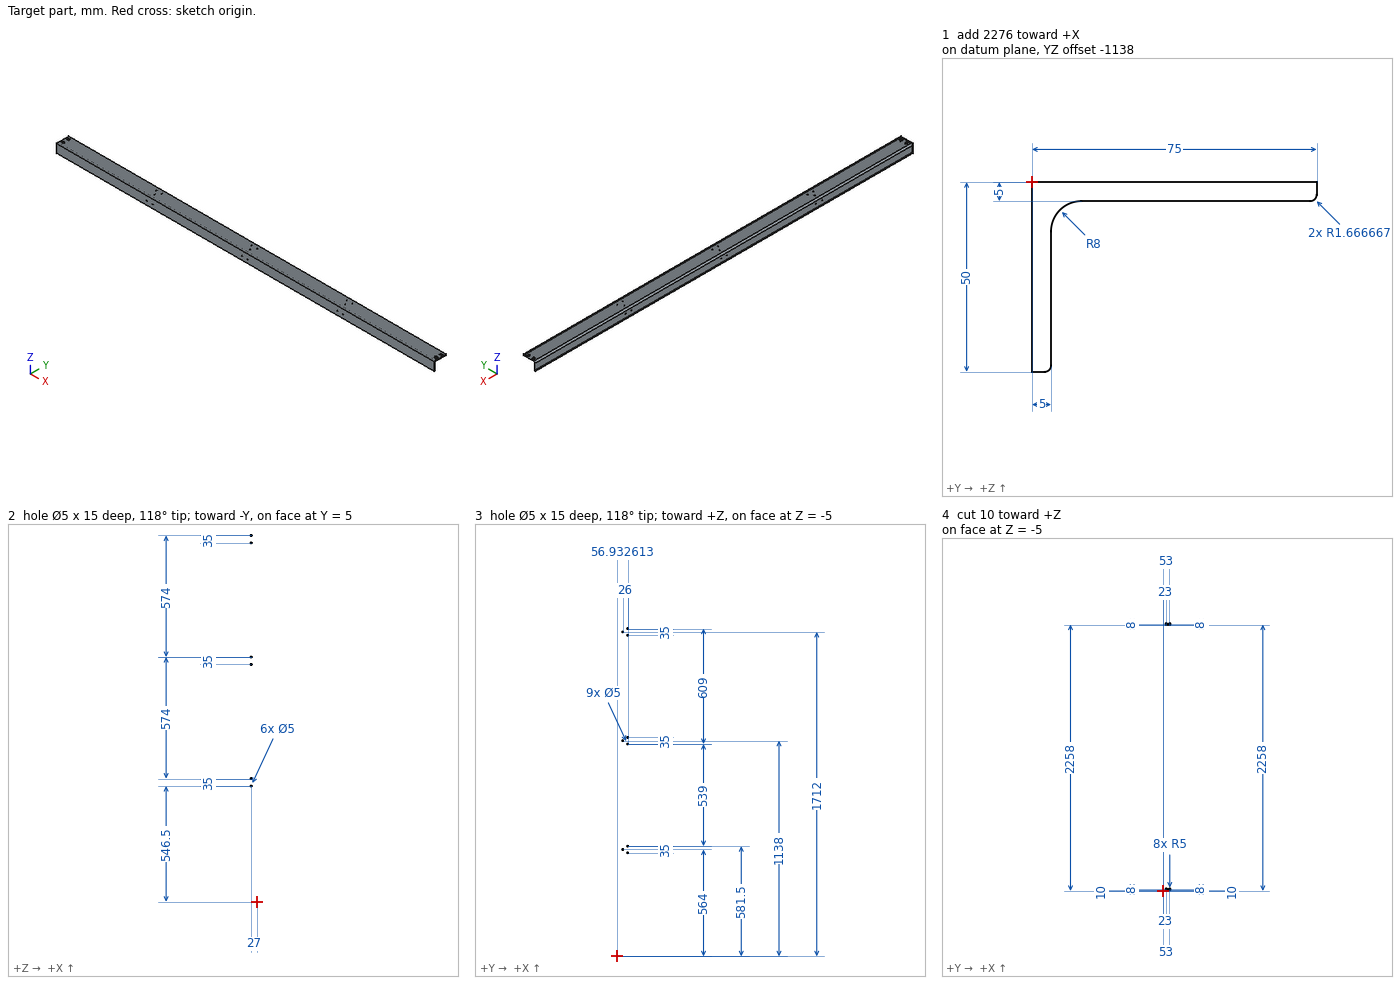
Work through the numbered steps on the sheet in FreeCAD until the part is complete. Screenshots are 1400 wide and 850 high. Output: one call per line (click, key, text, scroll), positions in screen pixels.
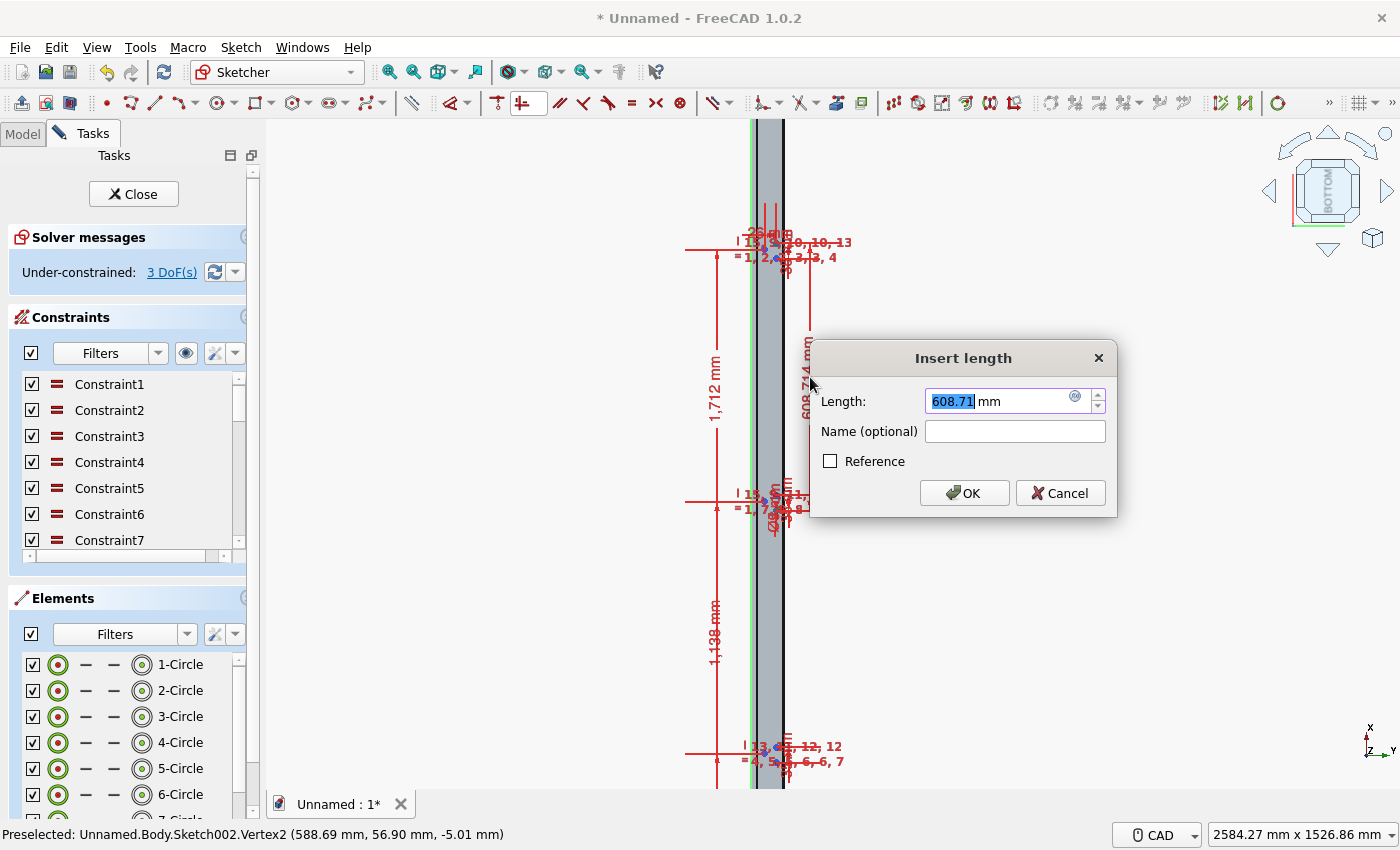
text(609)
key(Return)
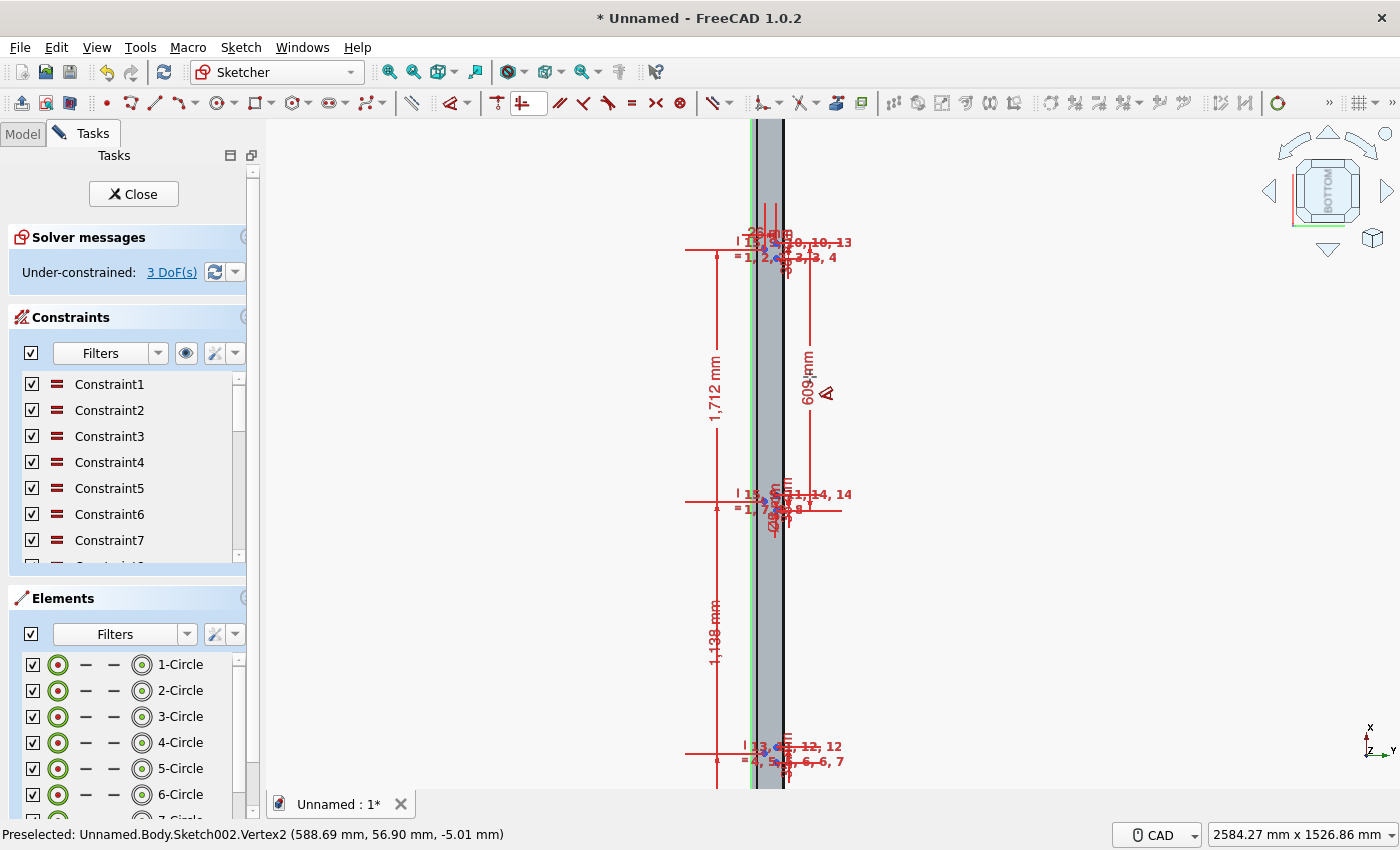
click(776, 511)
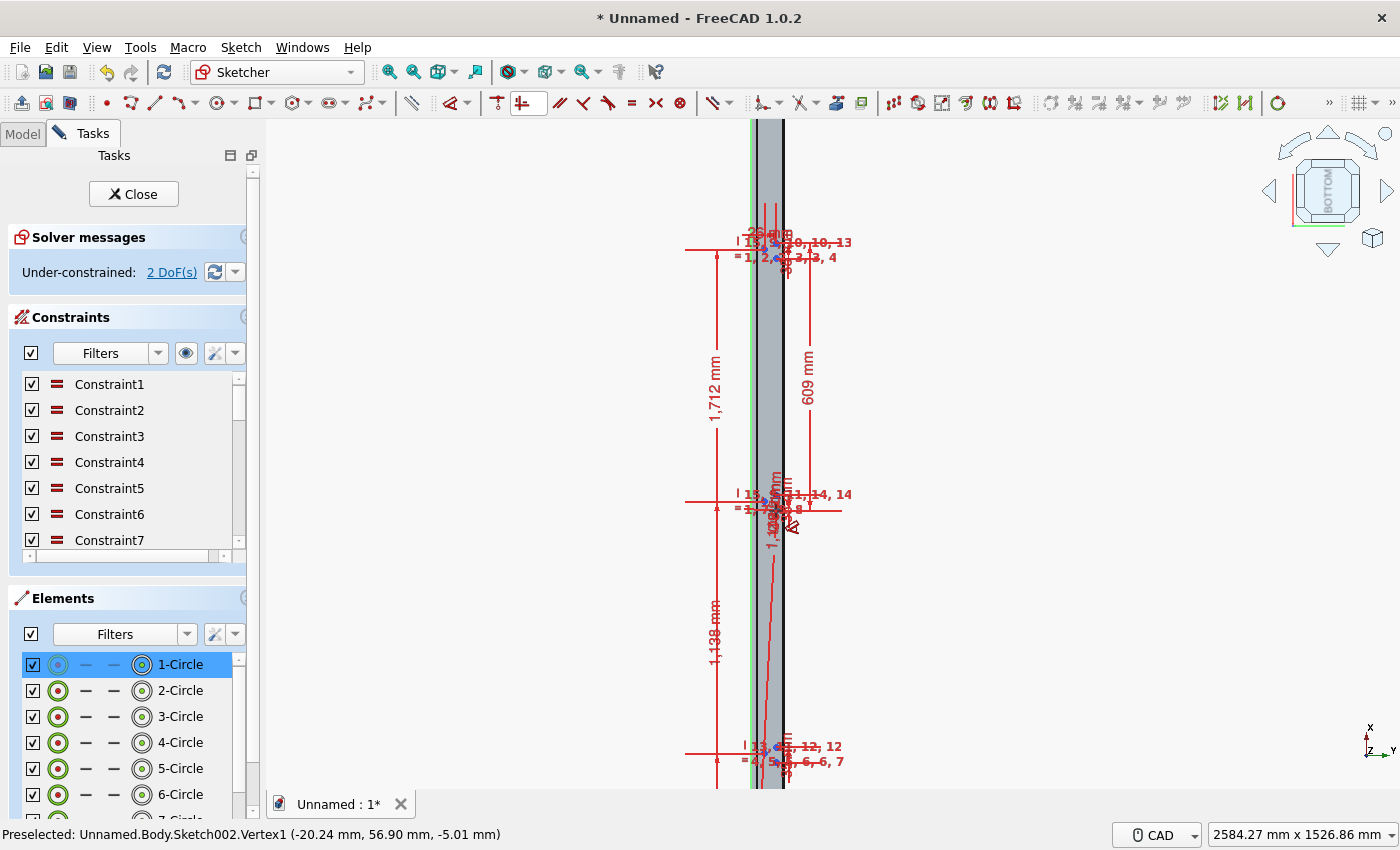
click(776, 747)
click(810, 629)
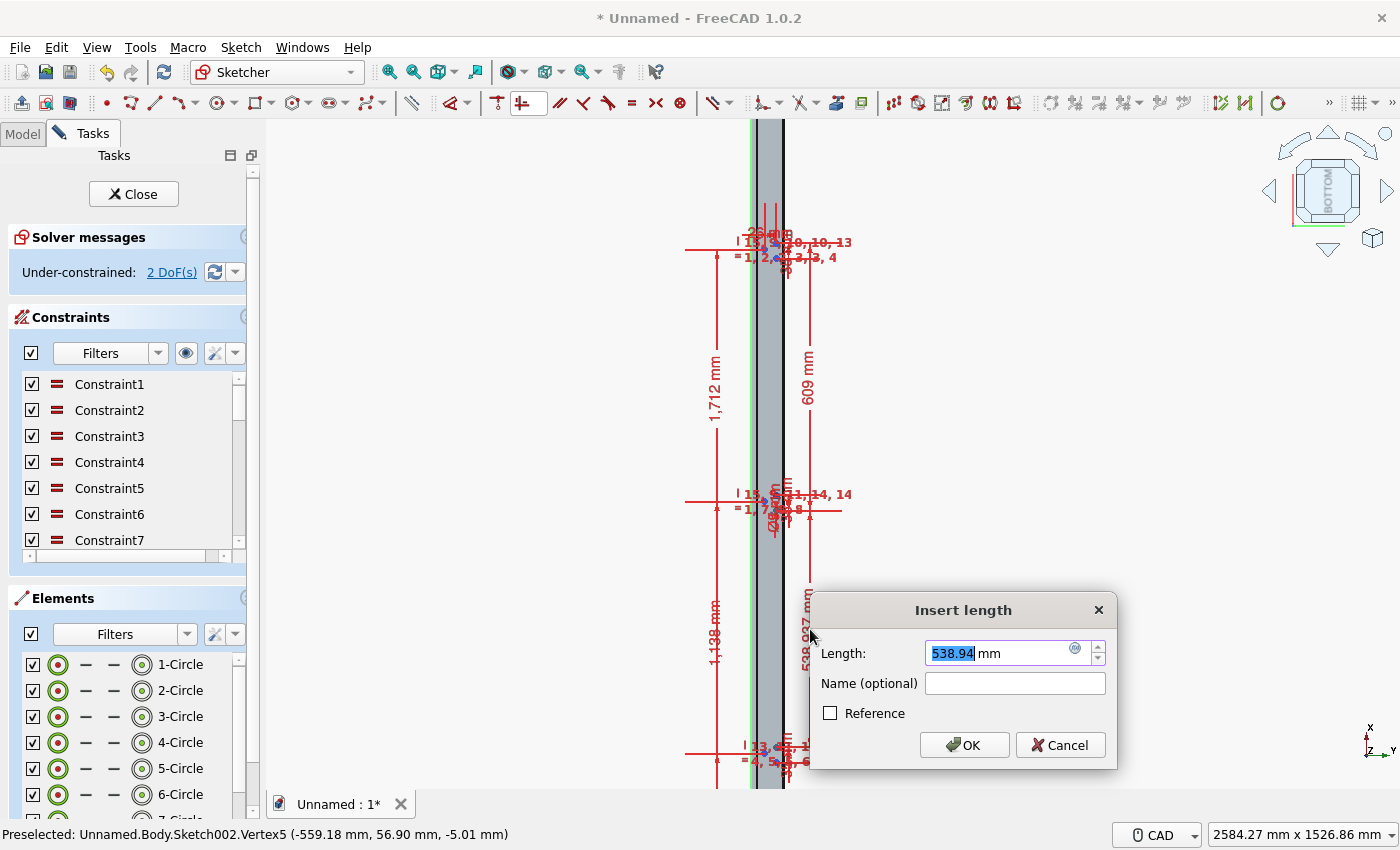
text(539)
key(Return)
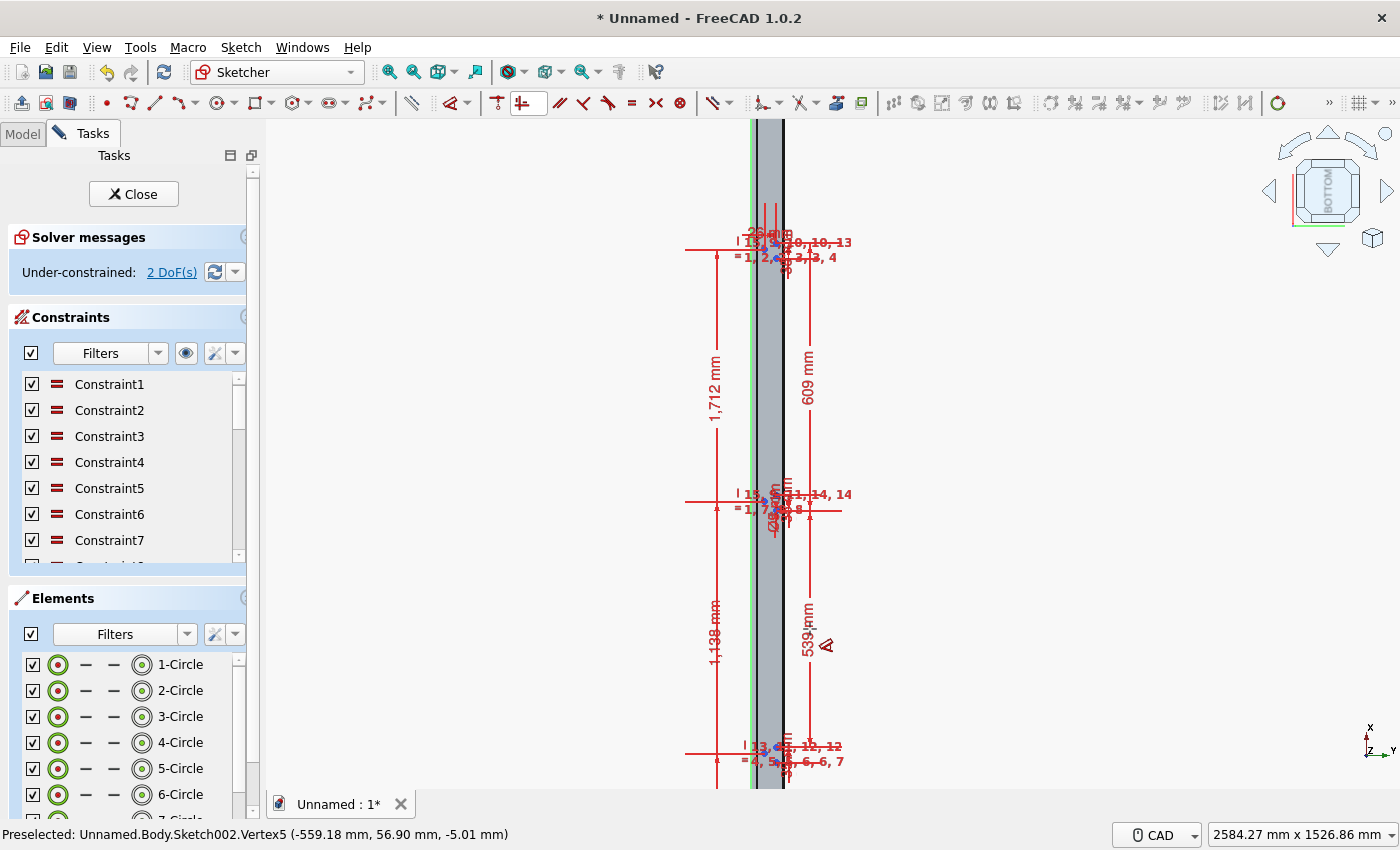
click(776, 747)
click(717, 754)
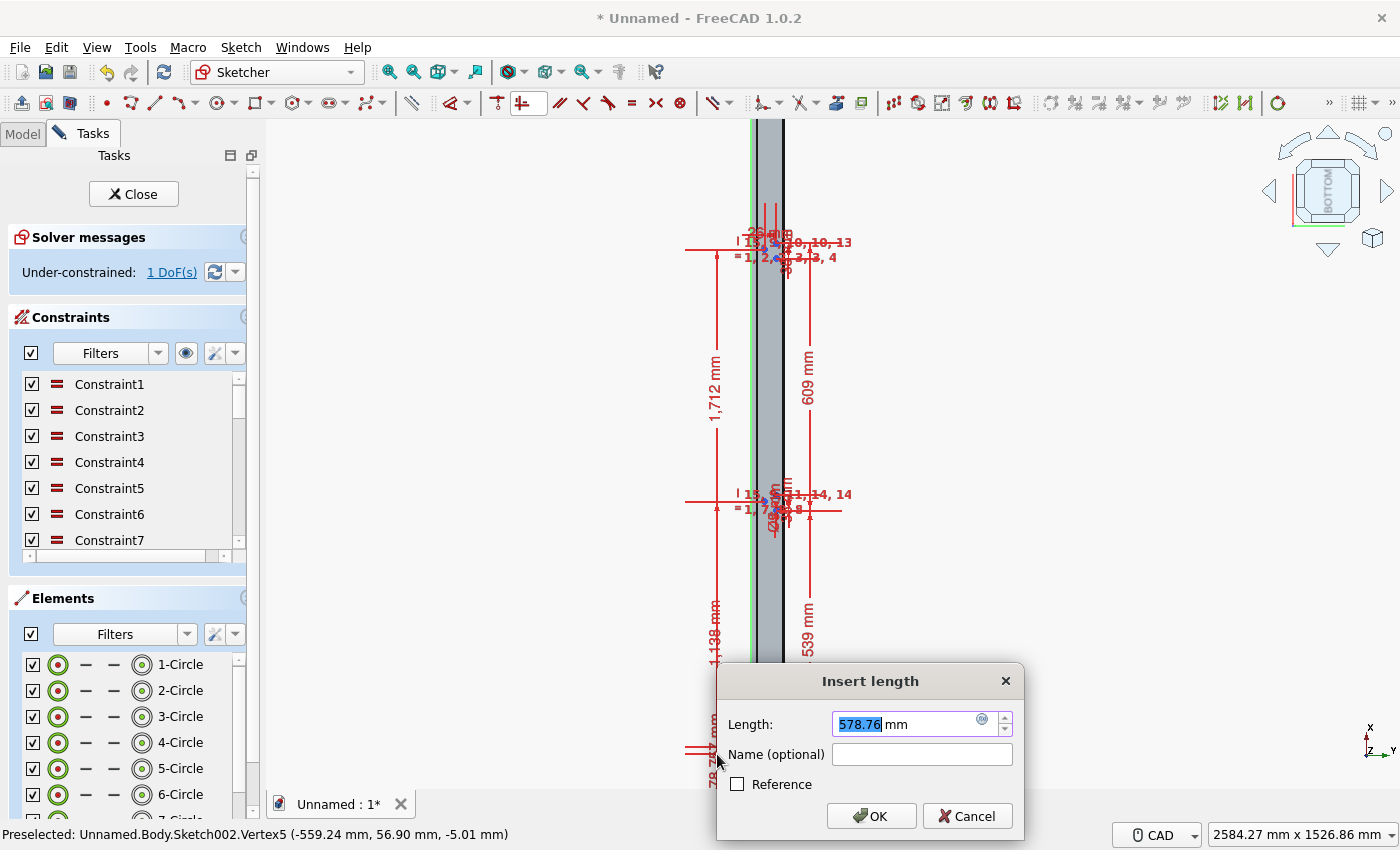
text(581.5)
key(Return)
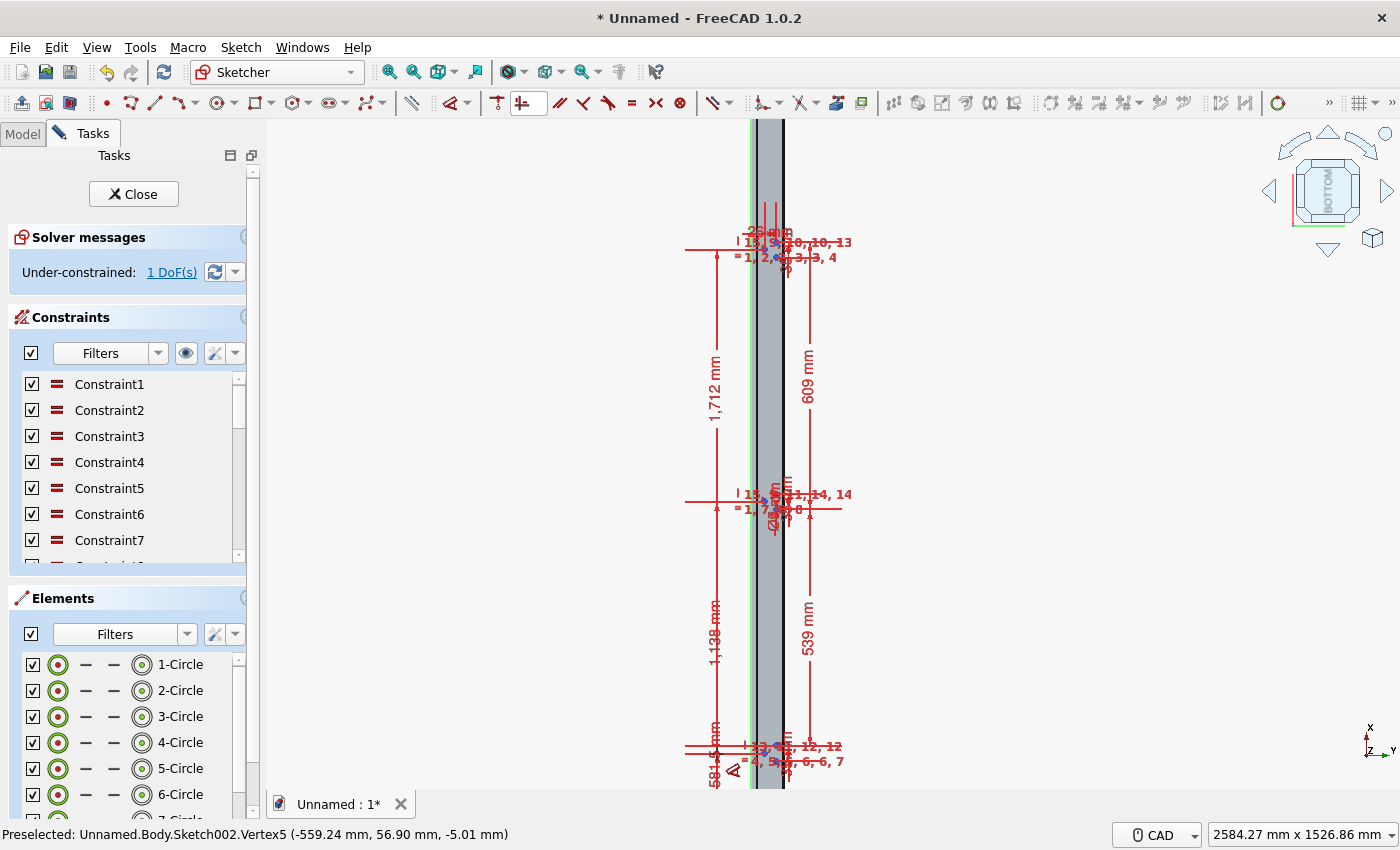
scroll(776, 509, up, 3)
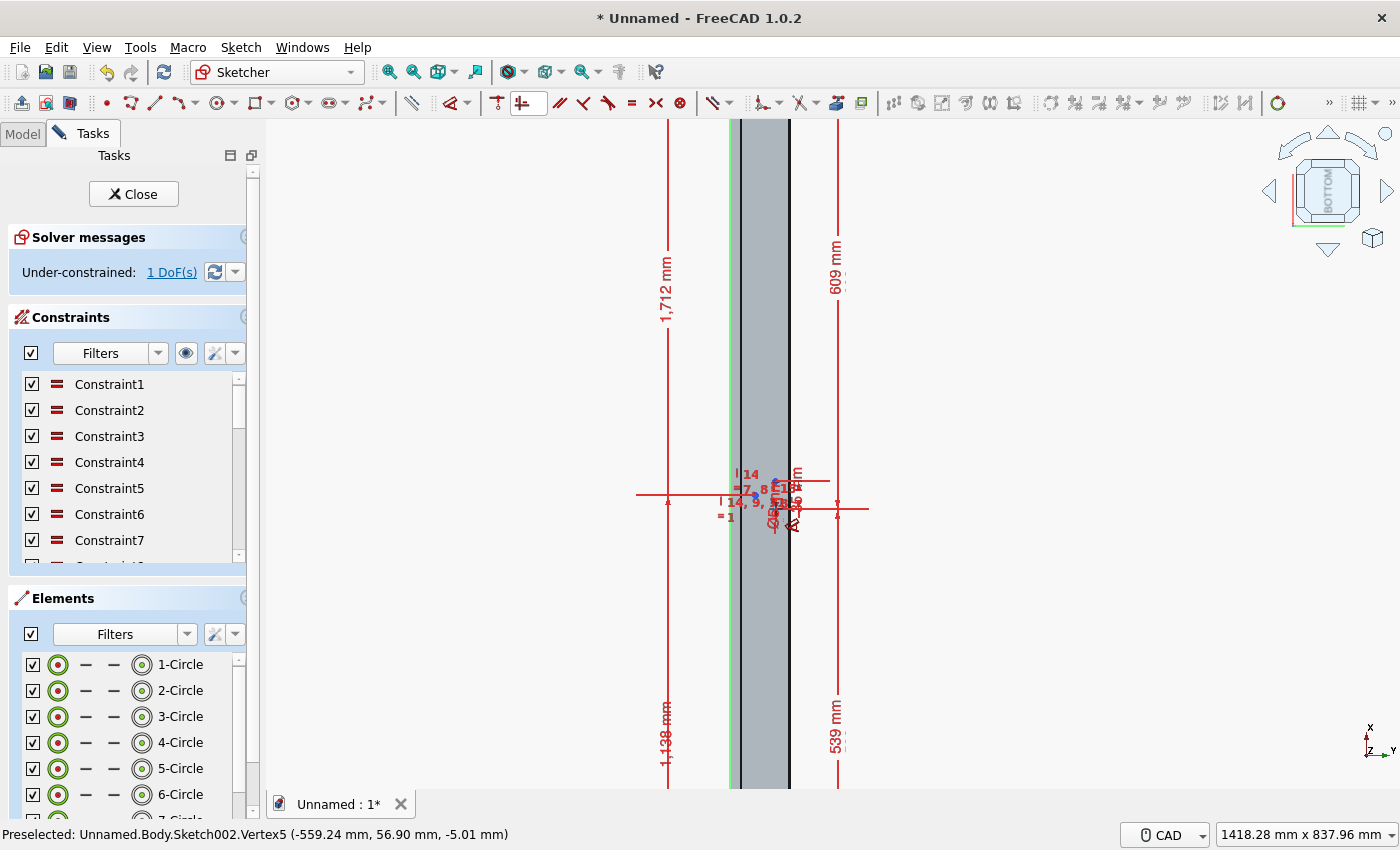
click(776, 509)
click(753, 451)